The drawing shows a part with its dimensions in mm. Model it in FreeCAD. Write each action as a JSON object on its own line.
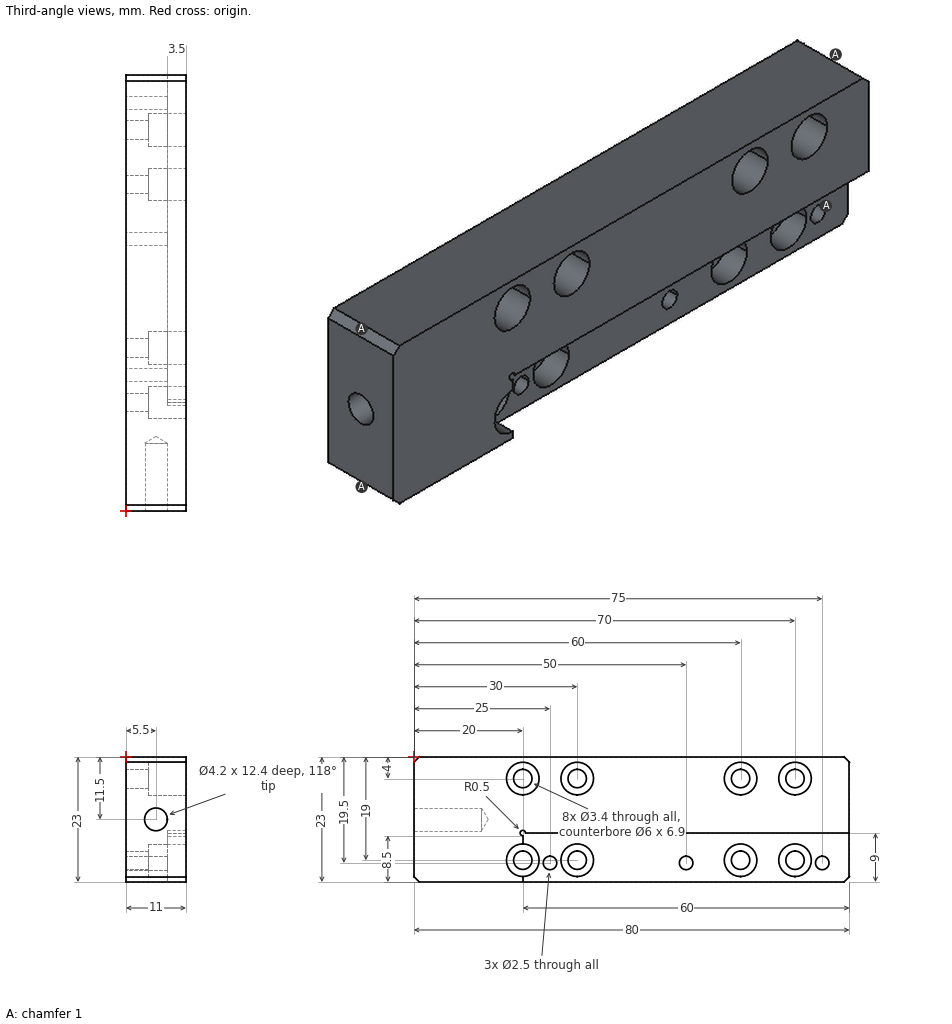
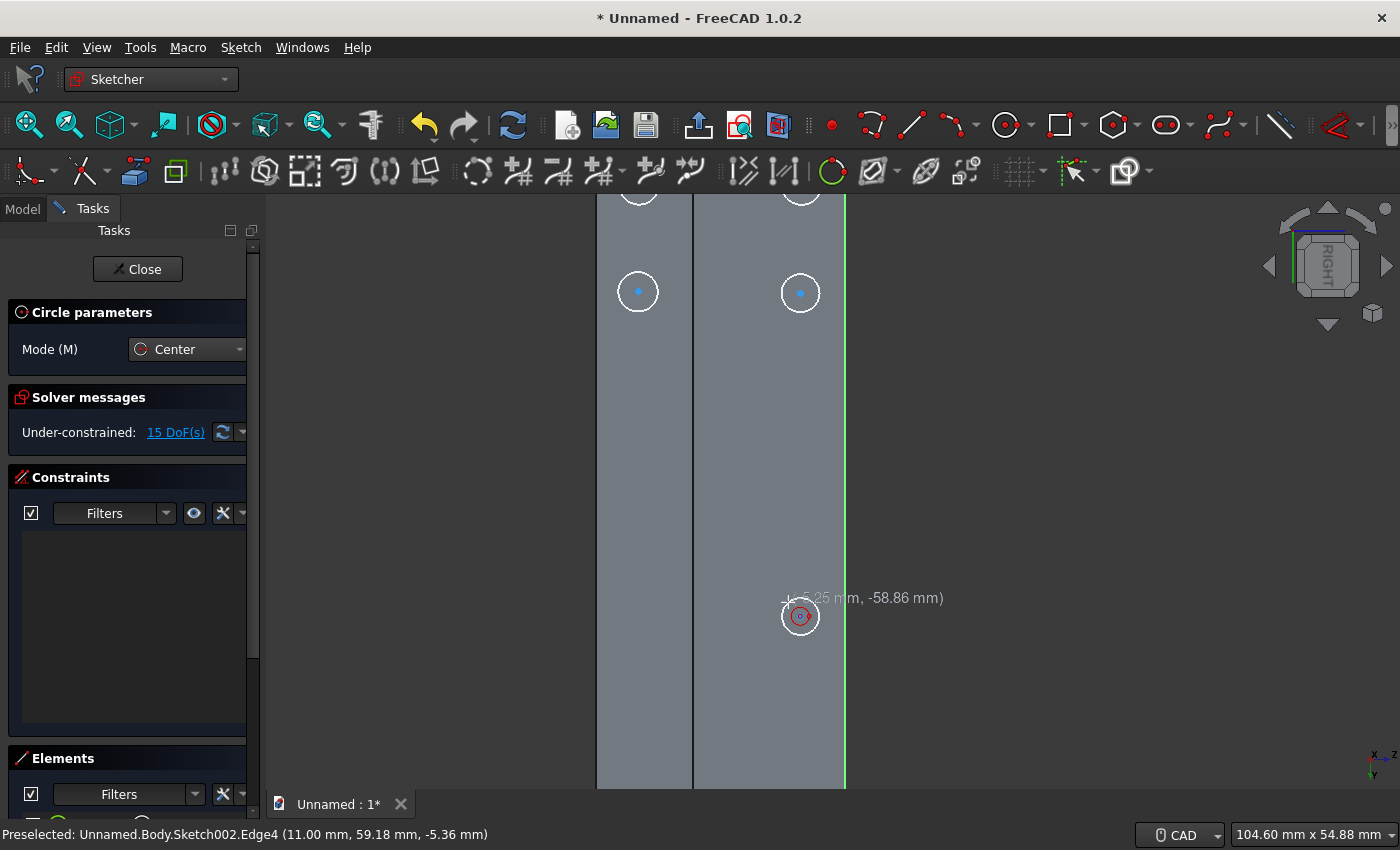
{"action": "scroll", "coordinate": [802, 724], "scroll_direction": "up", "scroll_amount": 2}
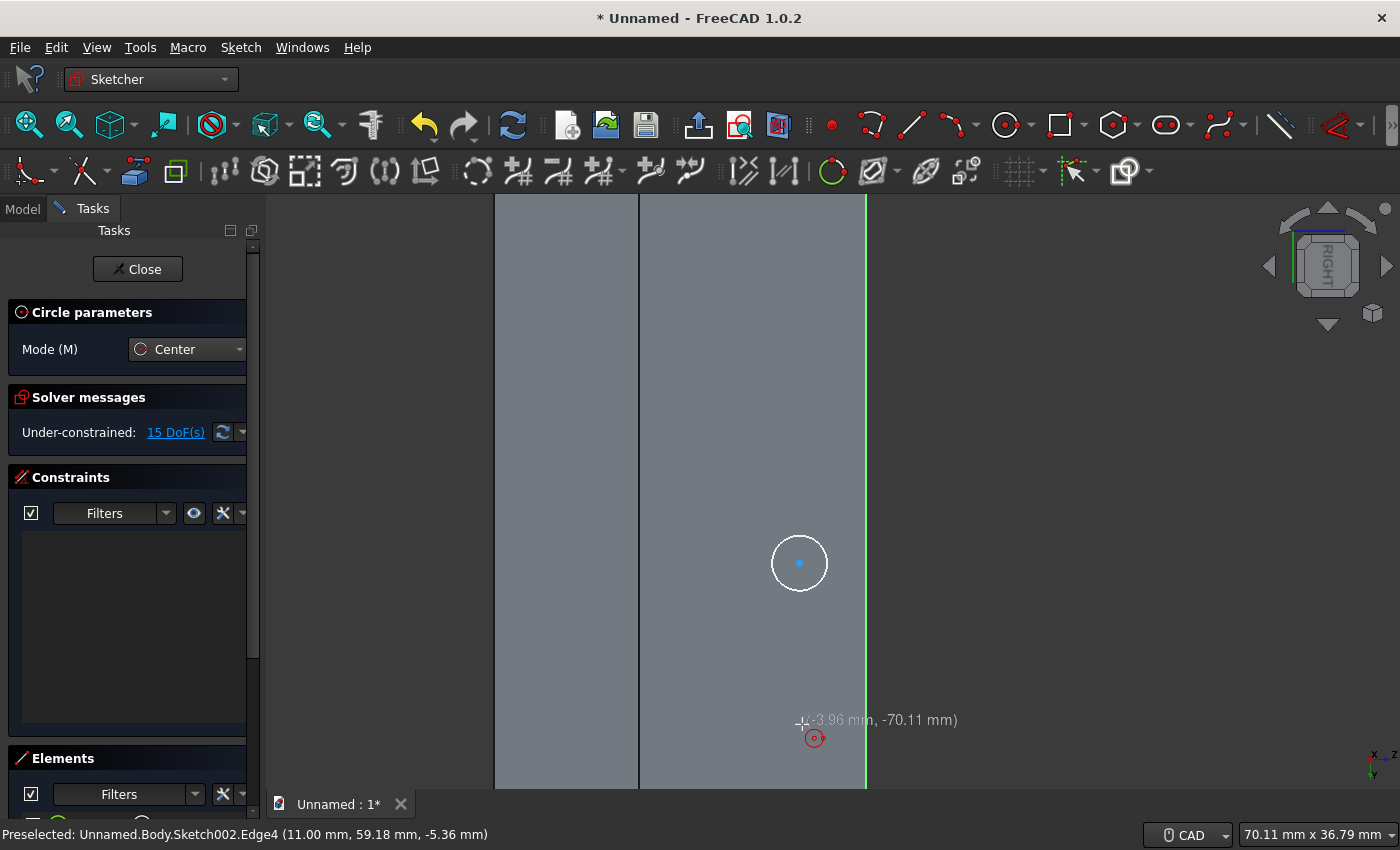
{"action": "scroll", "coordinate": [793, 630], "scroll_direction": "down", "scroll_amount": 6}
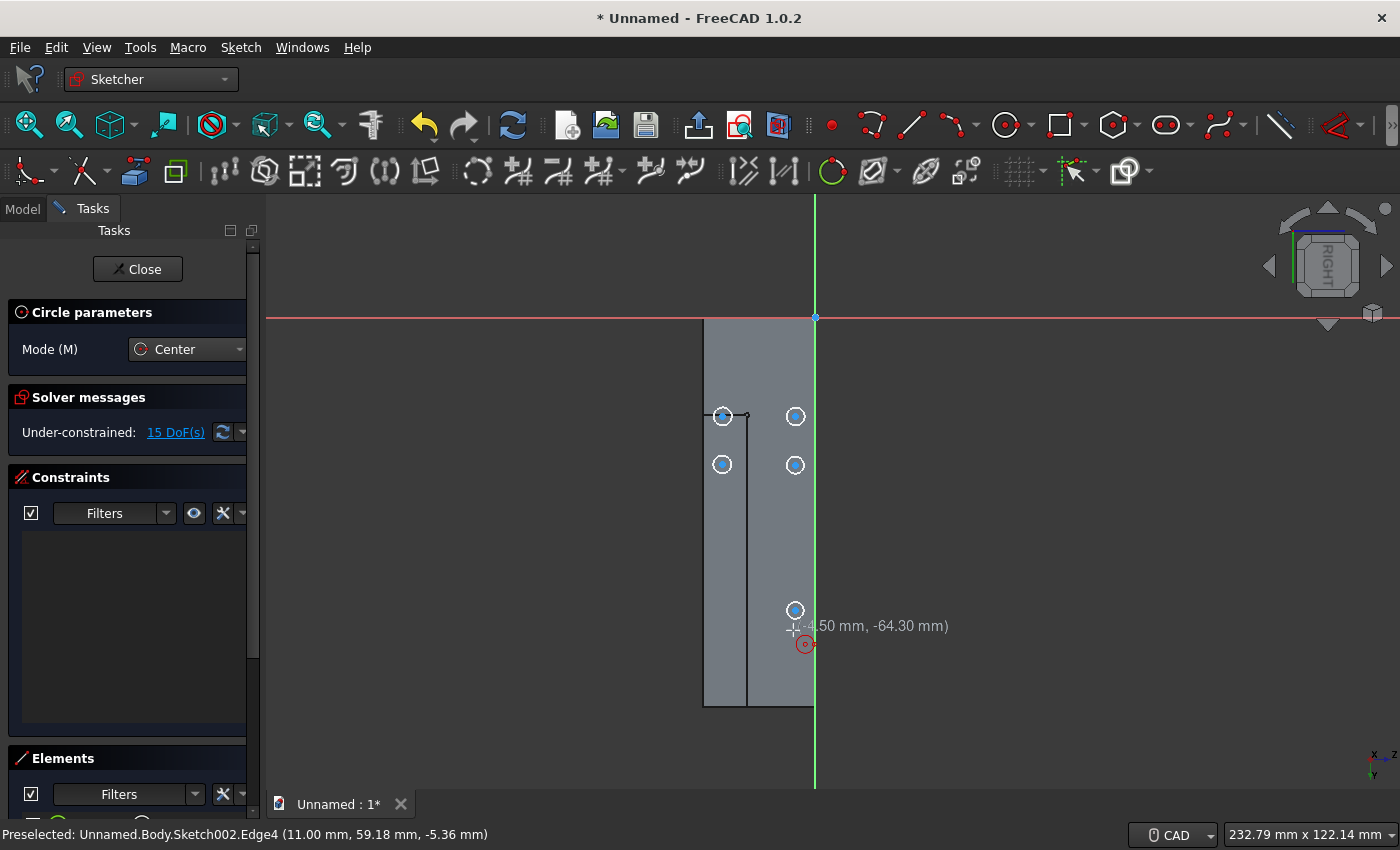
{"action": "left_click", "coordinate": [796, 659]}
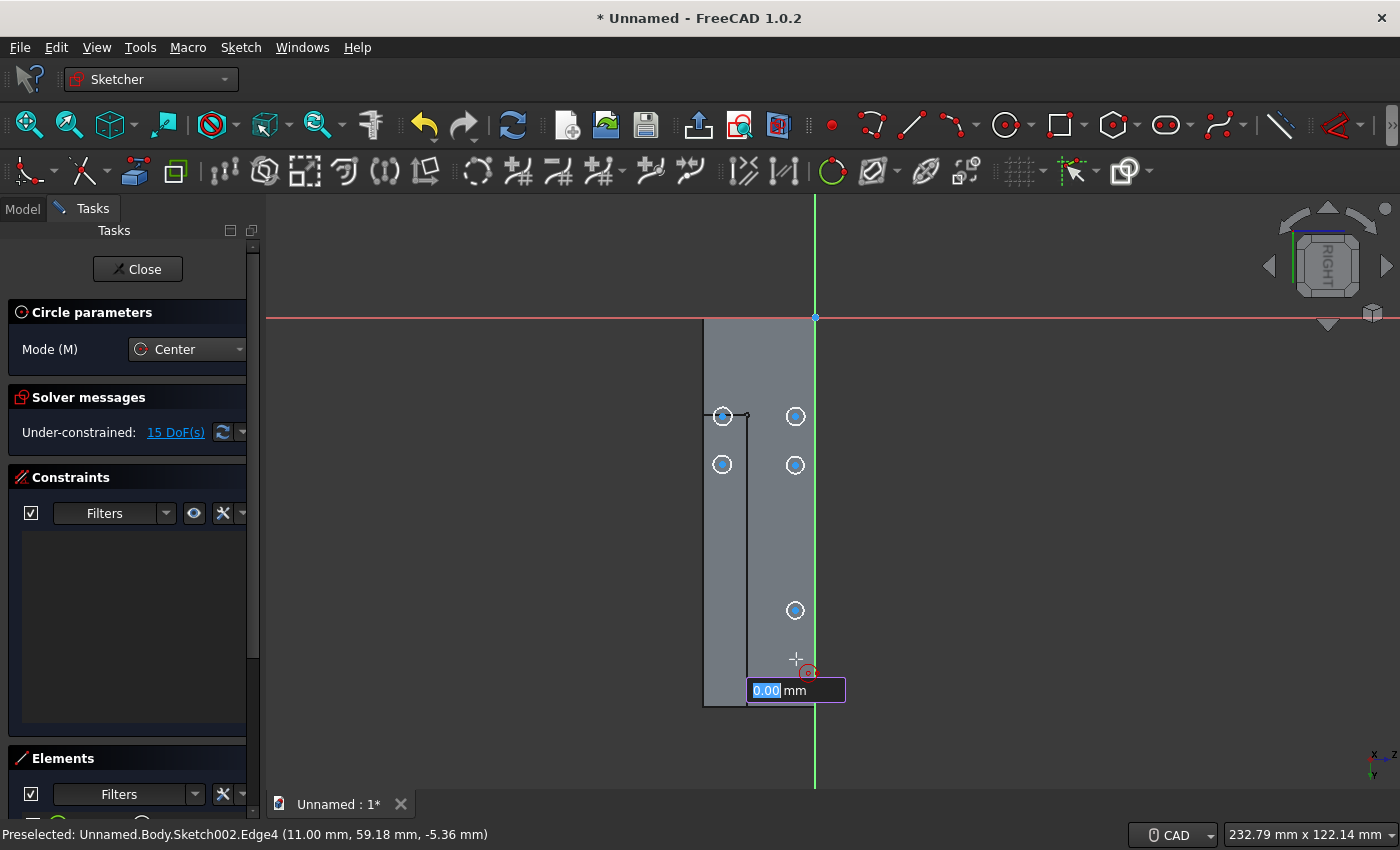
{"action": "scroll", "coordinate": [790, 653], "scroll_direction": "up", "scroll_amount": 4}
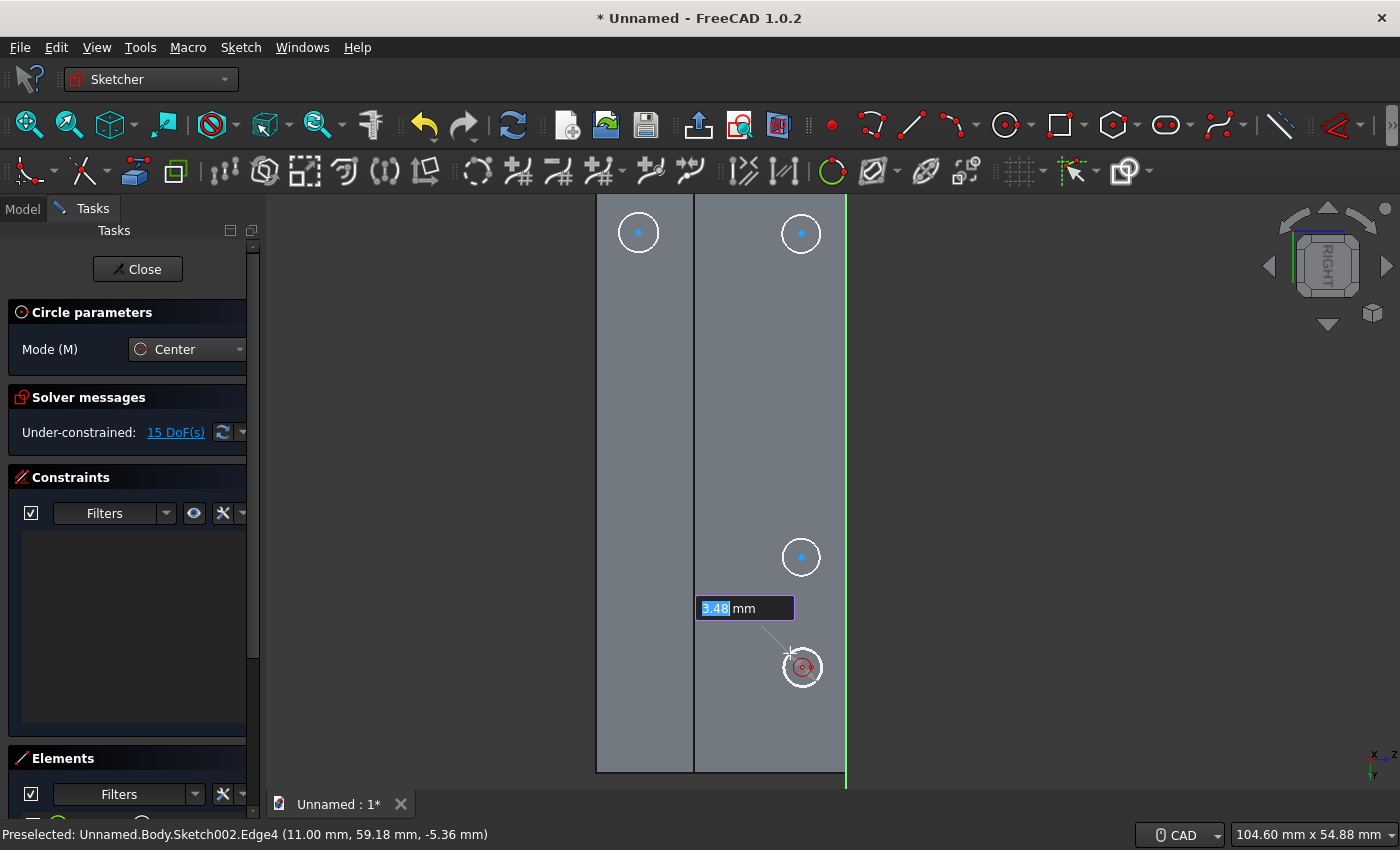
{"action": "left_click", "coordinate": [789, 651]}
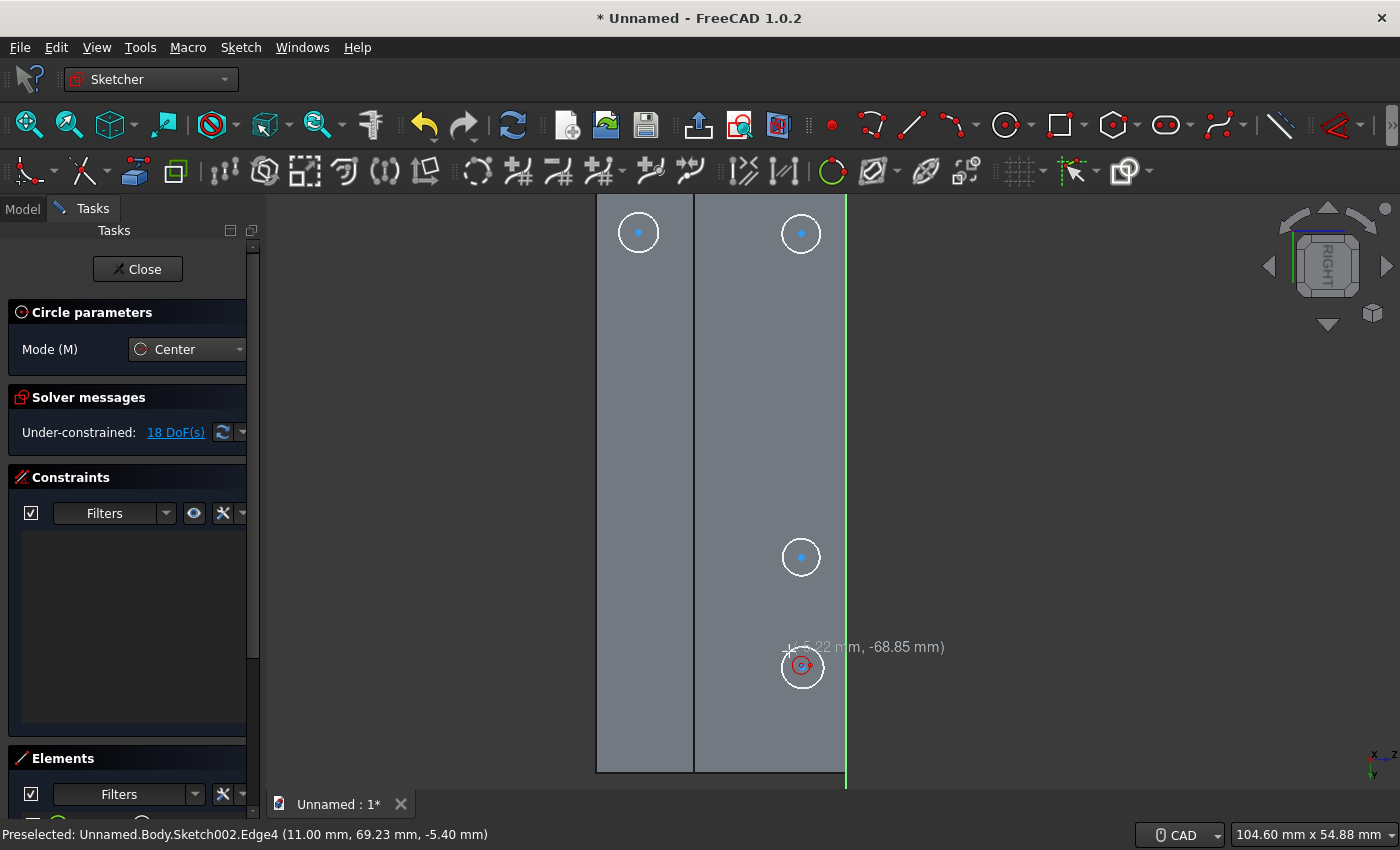
{"action": "scroll", "coordinate": [640, 556], "scroll_direction": "up", "scroll_amount": 2}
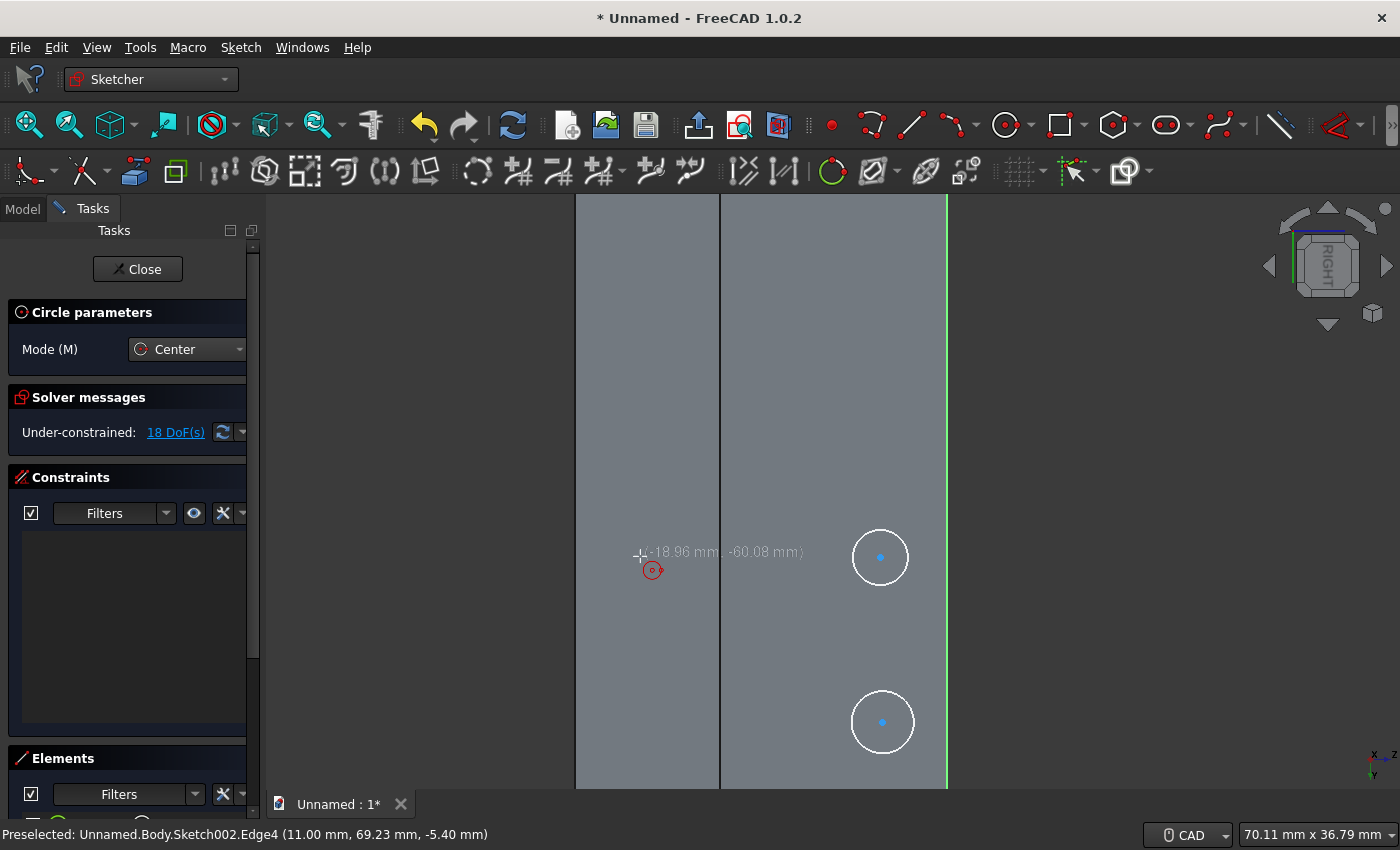
{"action": "scroll", "coordinate": [758, 632], "scroll_direction": "down", "scroll_amount": 6}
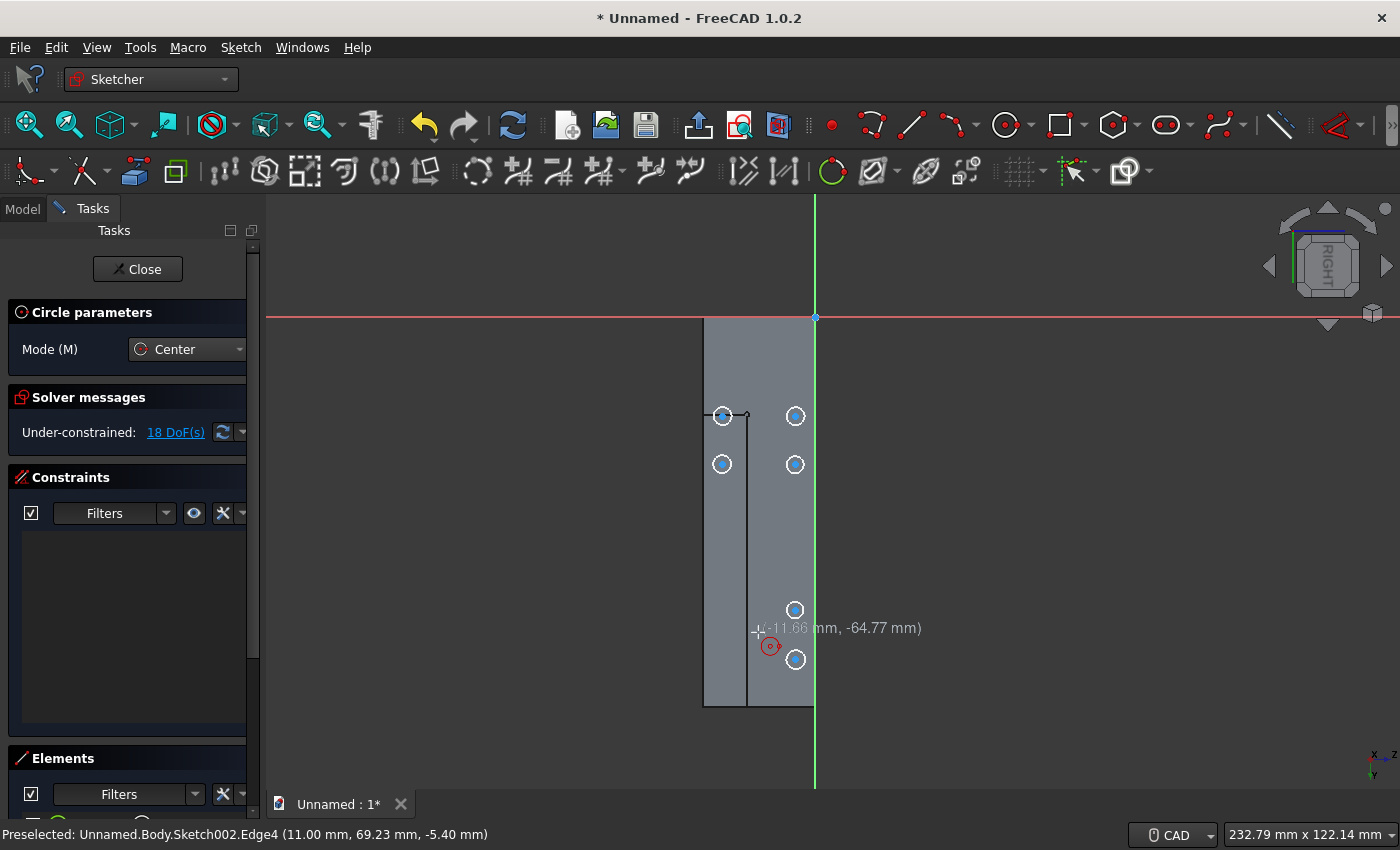
{"action": "left_click", "coordinate": [723, 610]}